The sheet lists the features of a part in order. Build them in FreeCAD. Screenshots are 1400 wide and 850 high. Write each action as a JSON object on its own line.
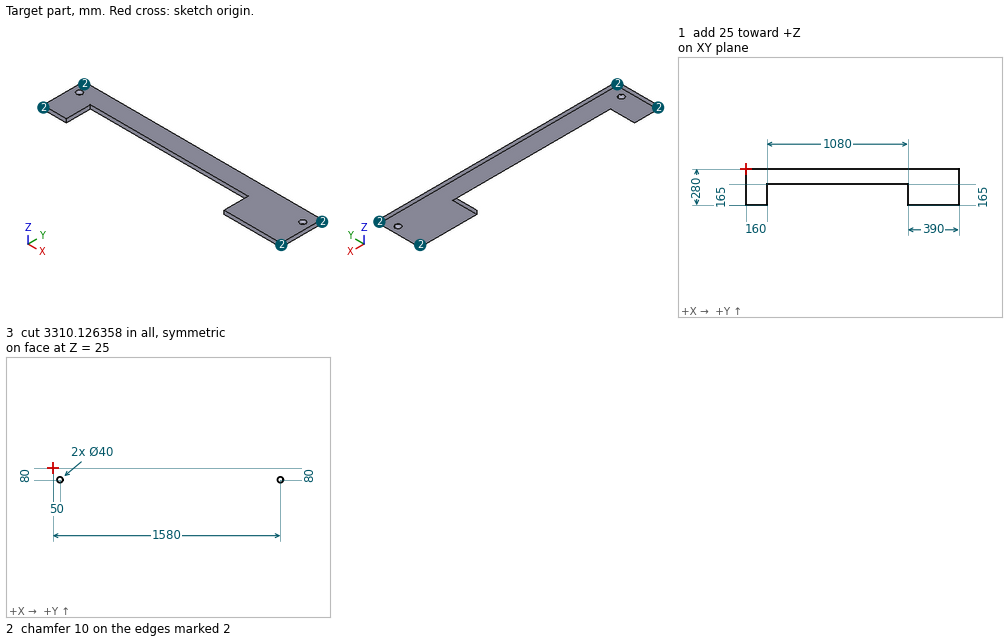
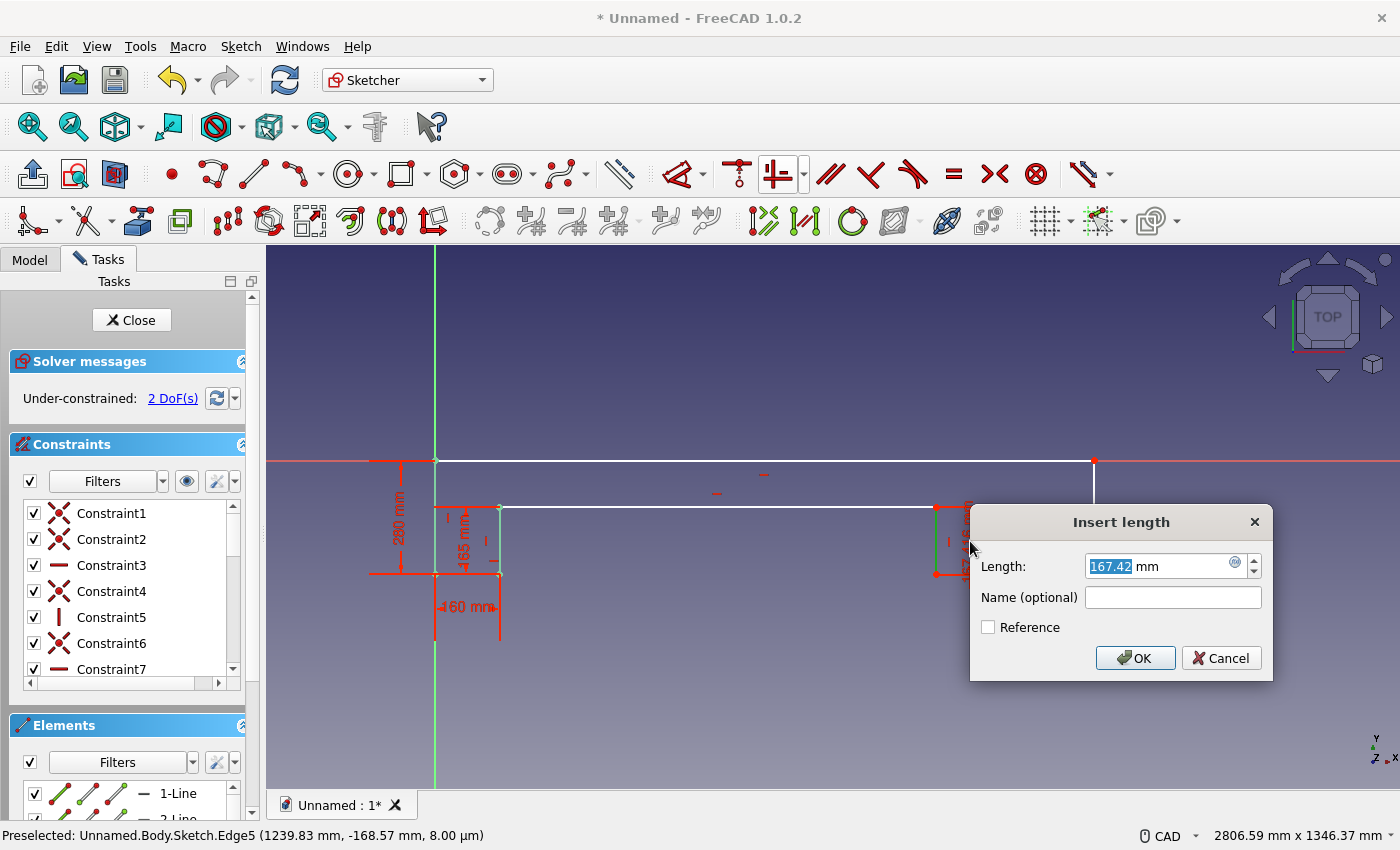
{"action": "type", "text": "165"}
{"action": "key", "text": "Return"}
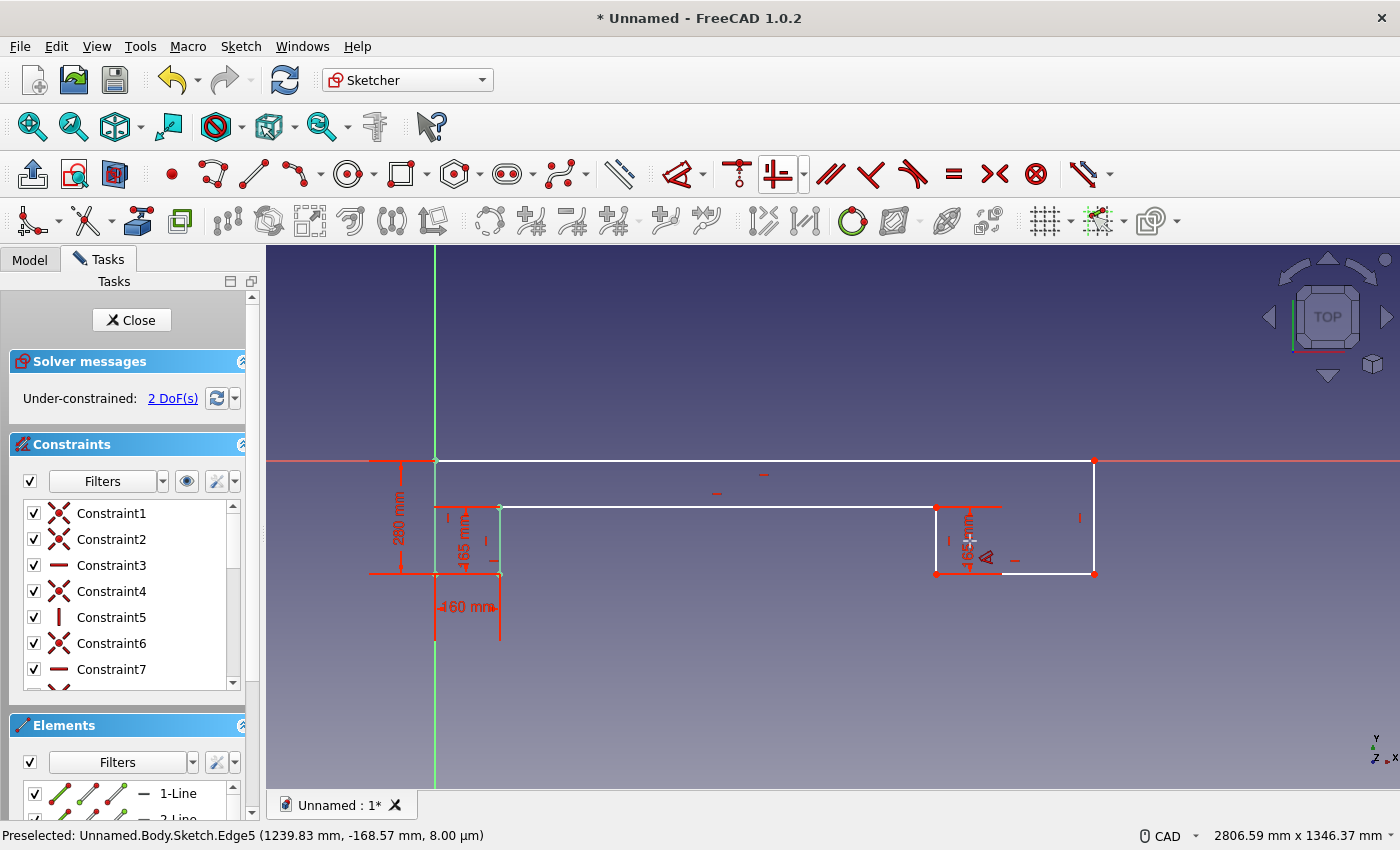
{"action": "left_click", "coordinate": [983, 574]}
{"action": "left_click", "coordinate": [1015, 608]}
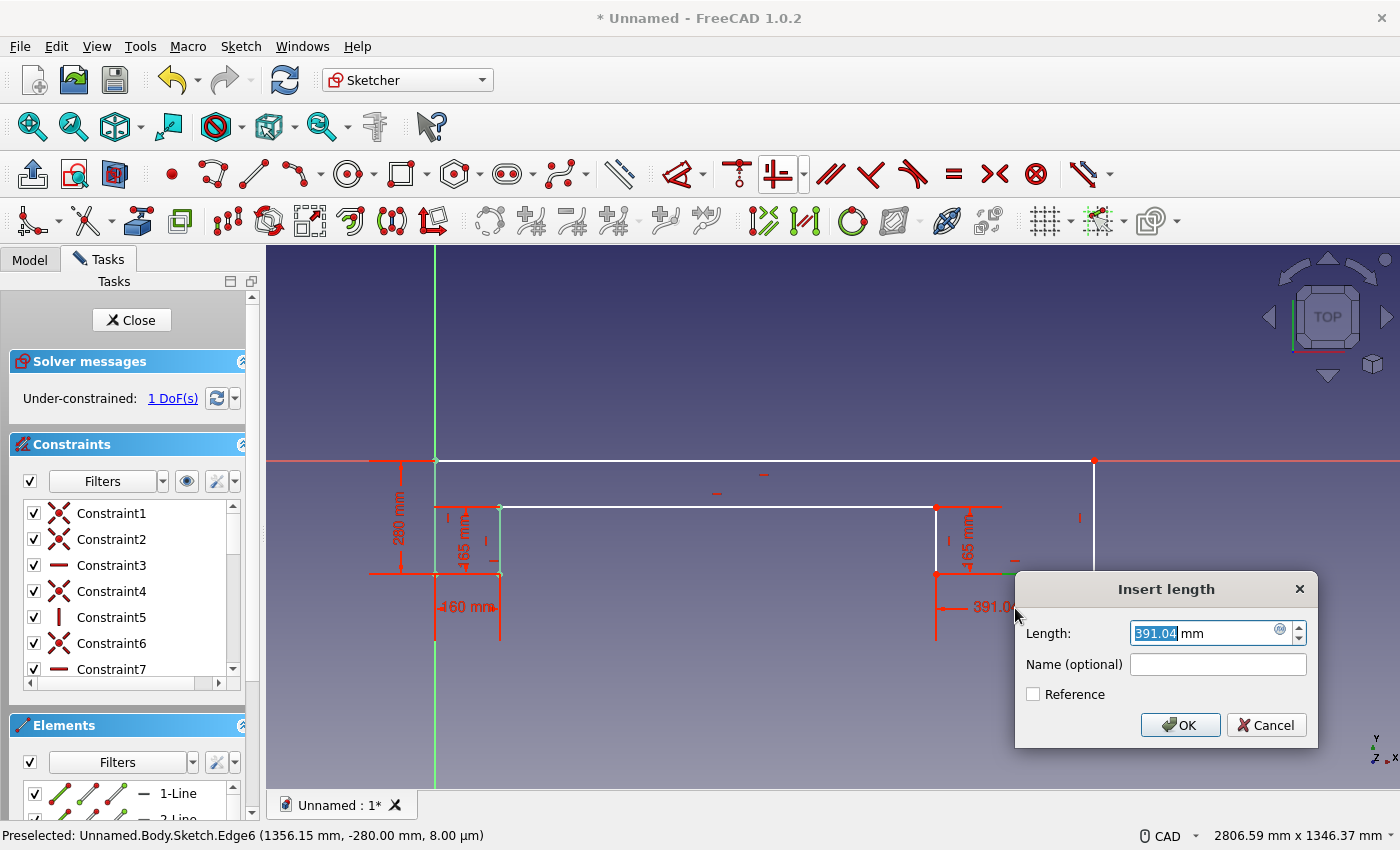
{"action": "type", "text": "390"}
{"action": "key", "text": "Return"}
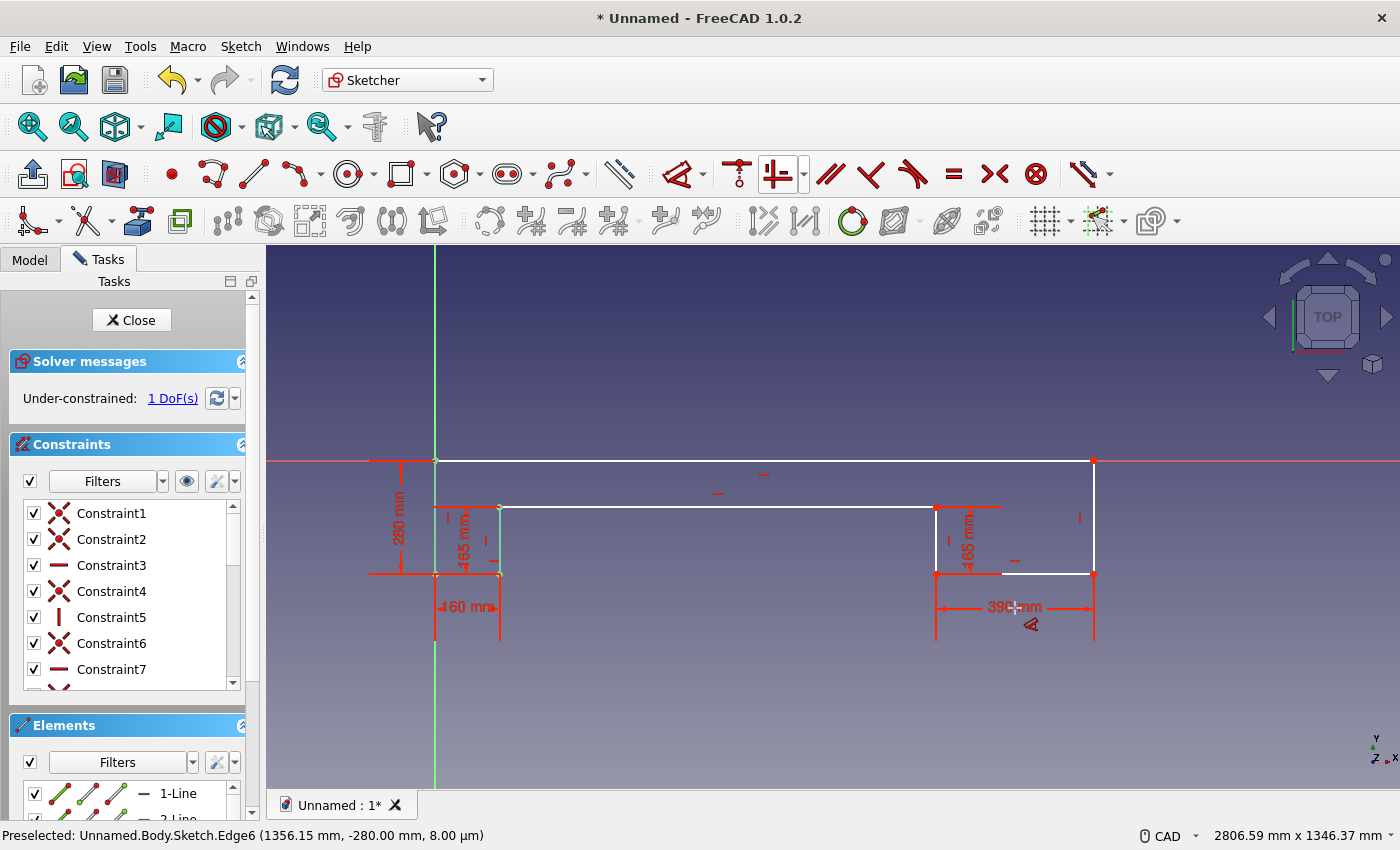
{"action": "left_click", "coordinate": [631, 507]}
{"action": "left_click", "coordinate": [718, 541]}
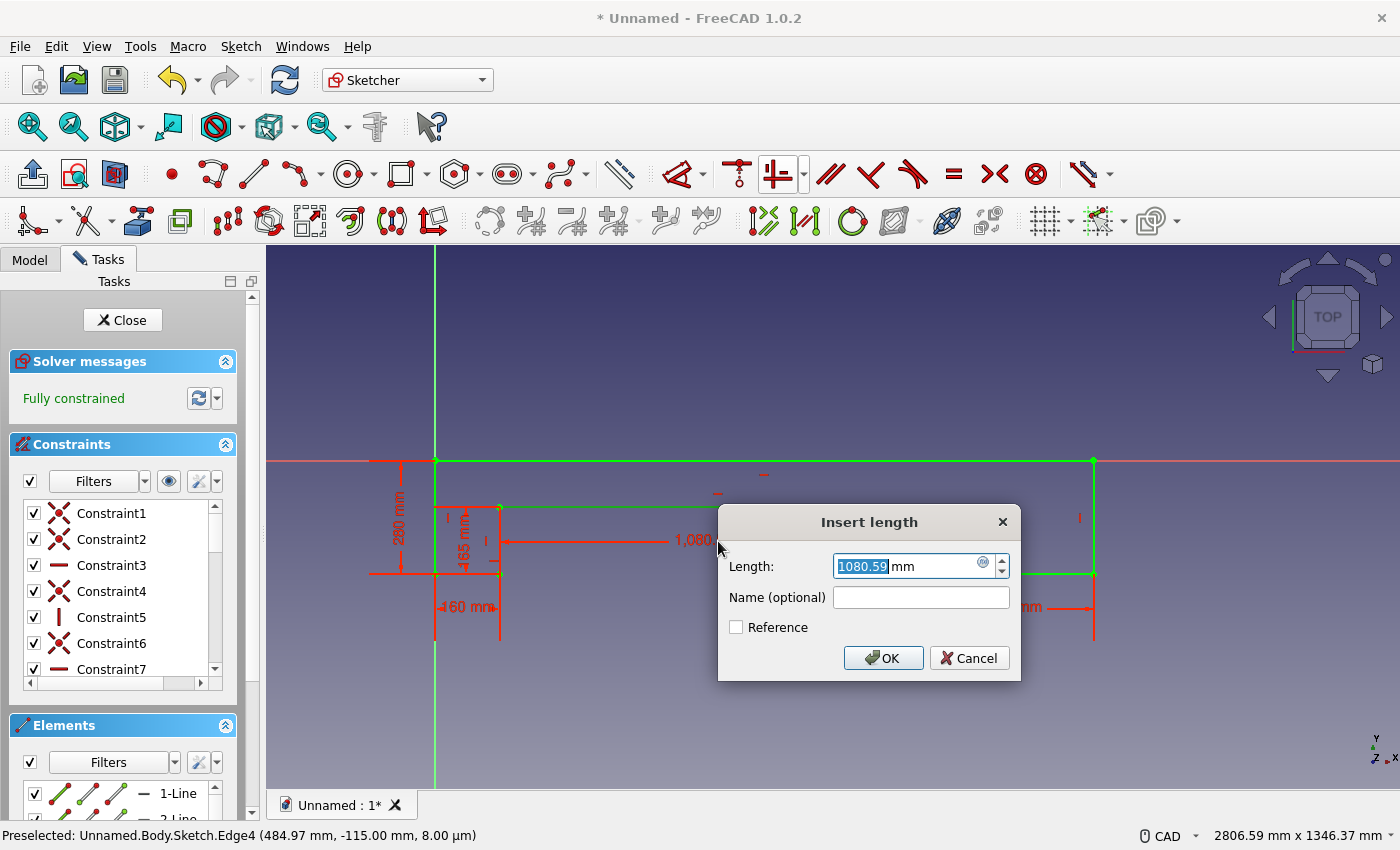
{"action": "type", "text": "1080"}
{"action": "key", "text": "Return"}
{"action": "key", "text": "Escape"}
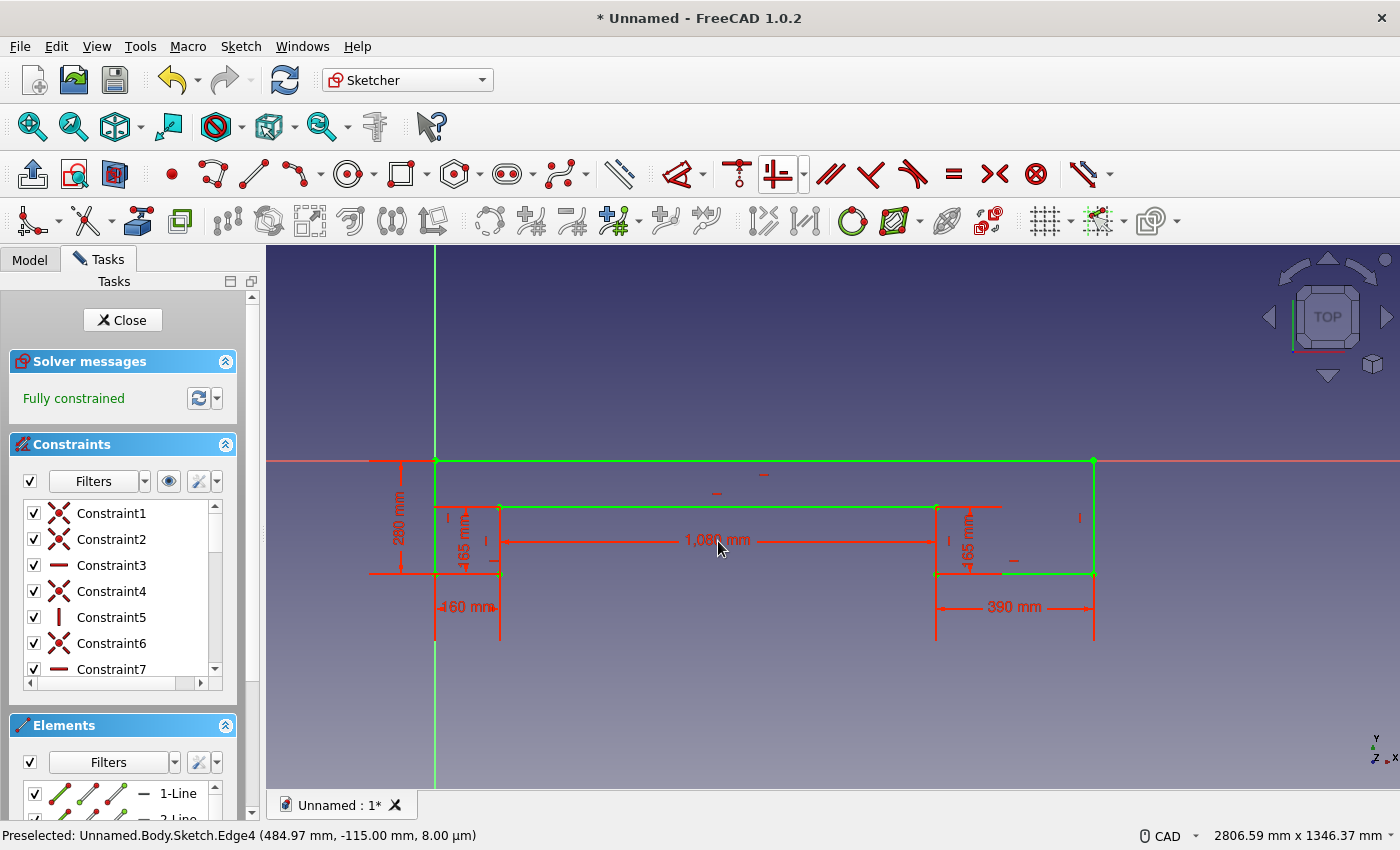
{"action": "left_click", "coordinate": [123, 320]}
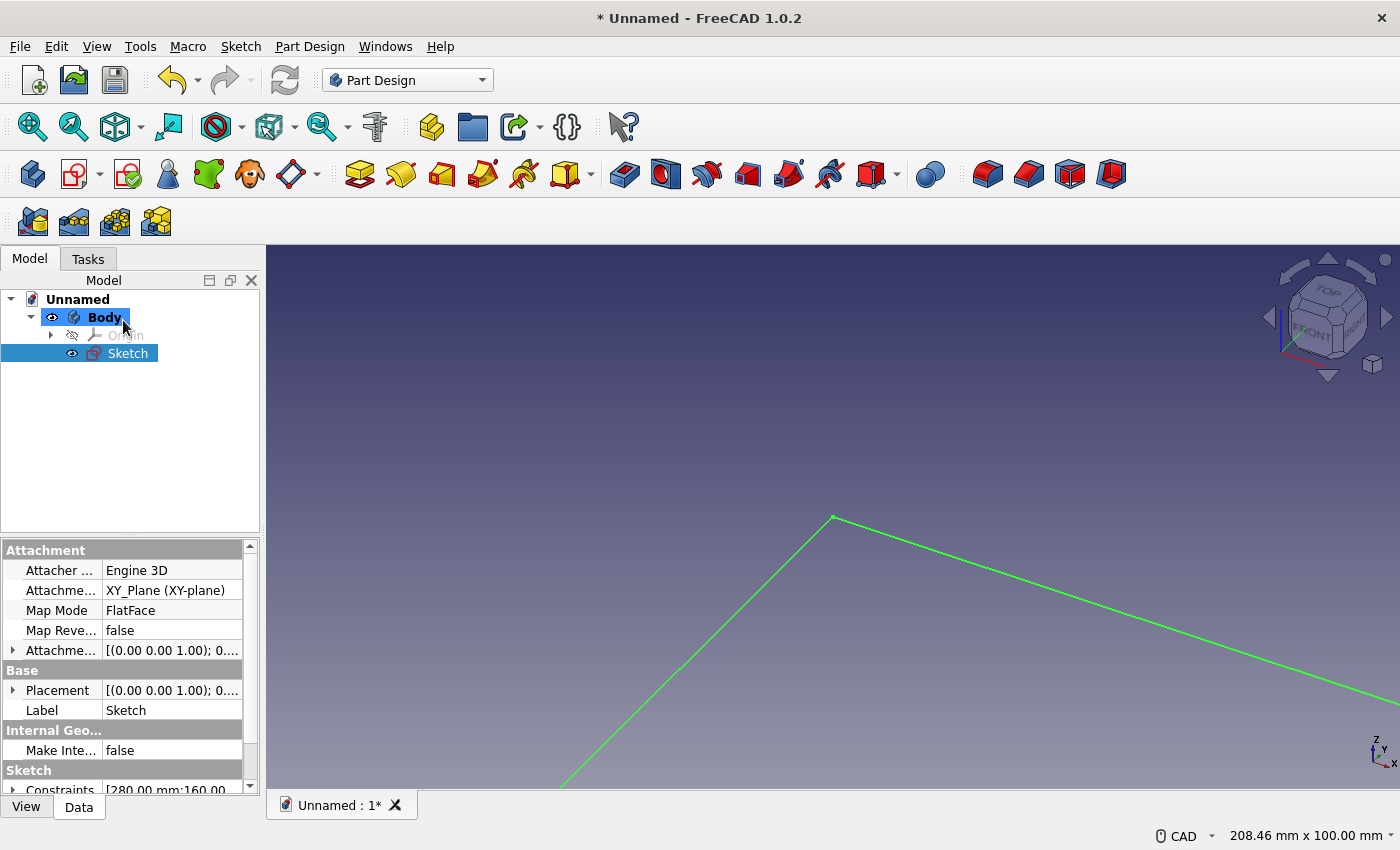
{"action": "left_click", "coordinate": [360, 174]}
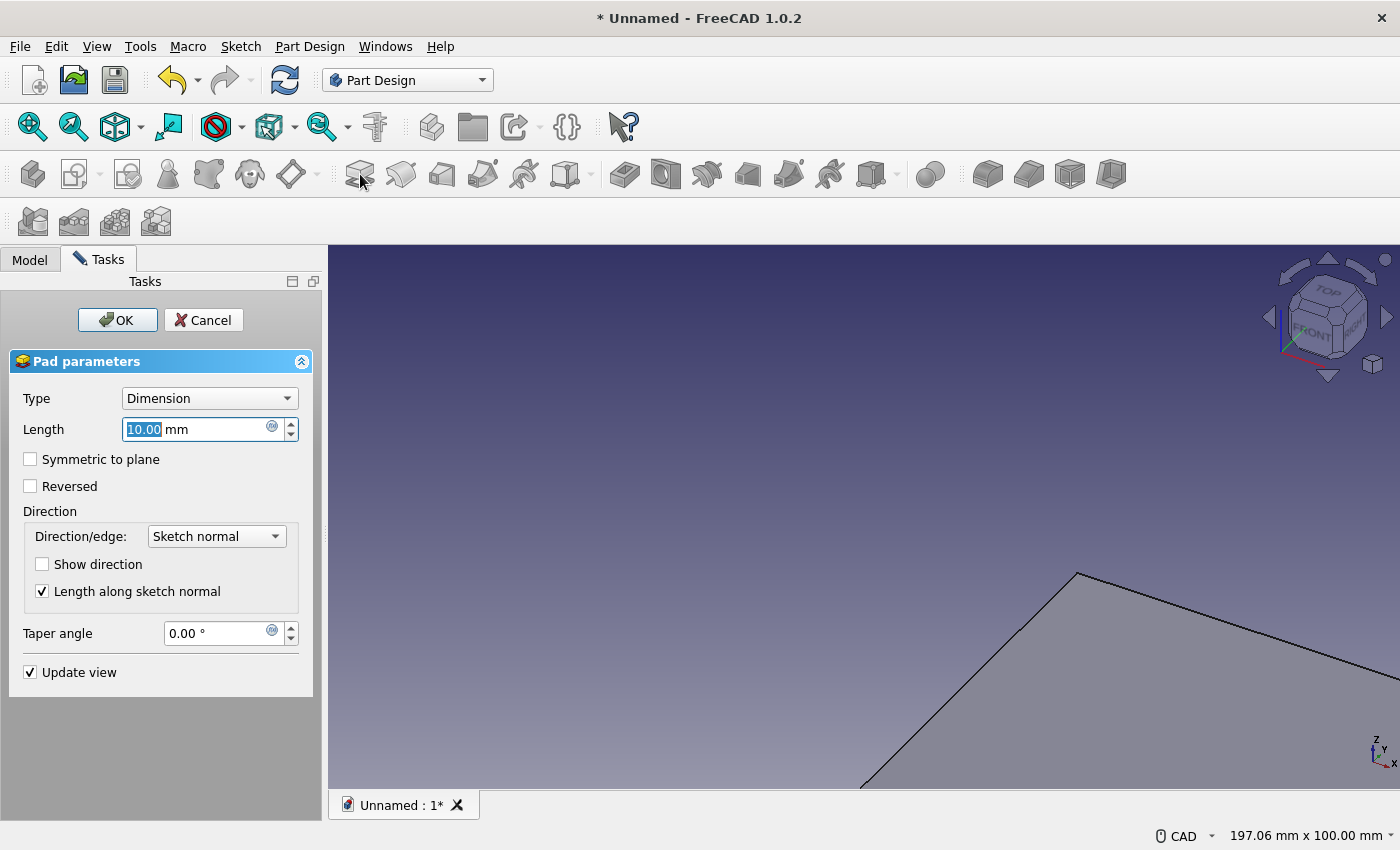
{"action": "type", "text": "25"}
{"action": "key", "text": "Tab"}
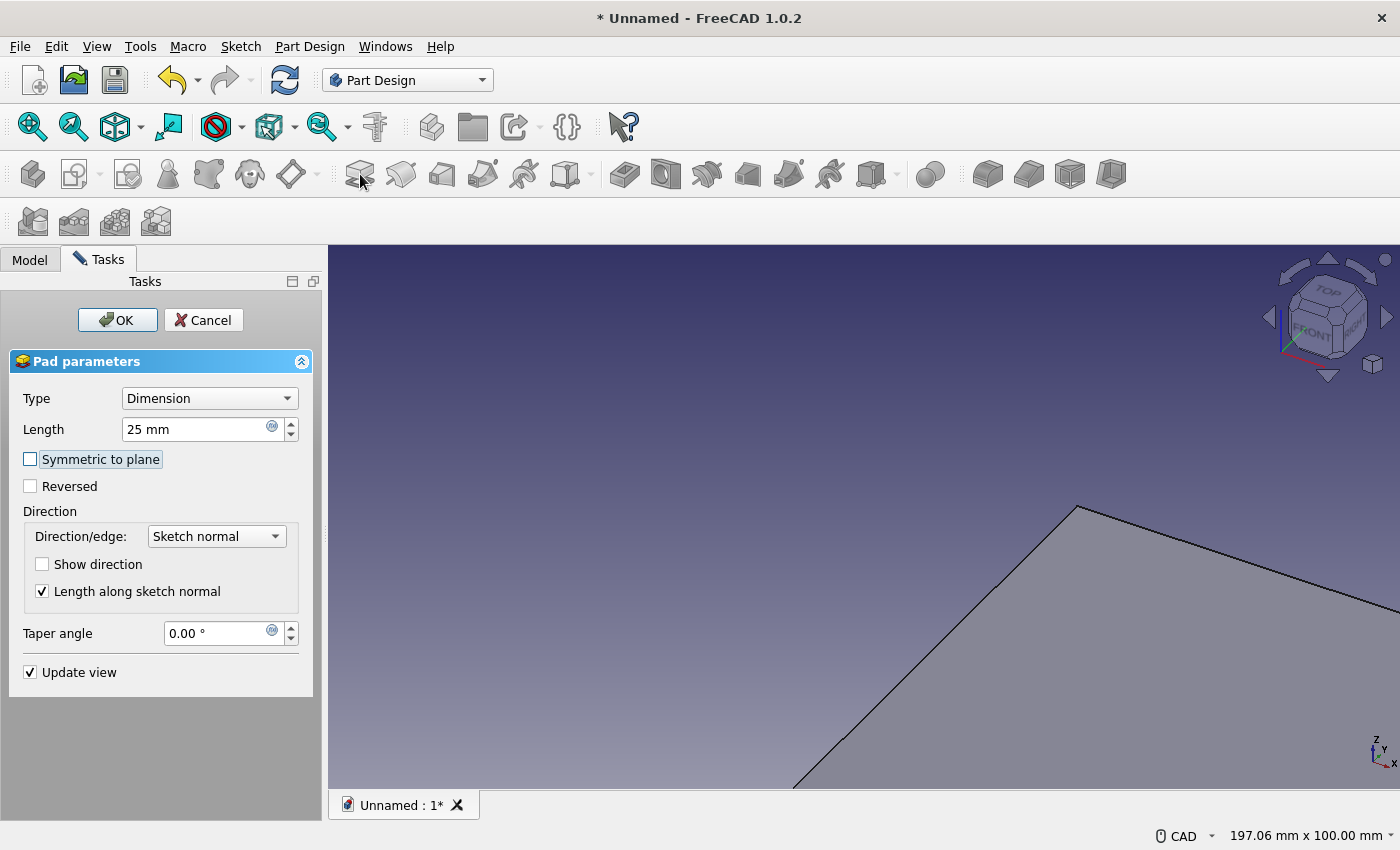
{"action": "left_click", "coordinate": [118, 320]}